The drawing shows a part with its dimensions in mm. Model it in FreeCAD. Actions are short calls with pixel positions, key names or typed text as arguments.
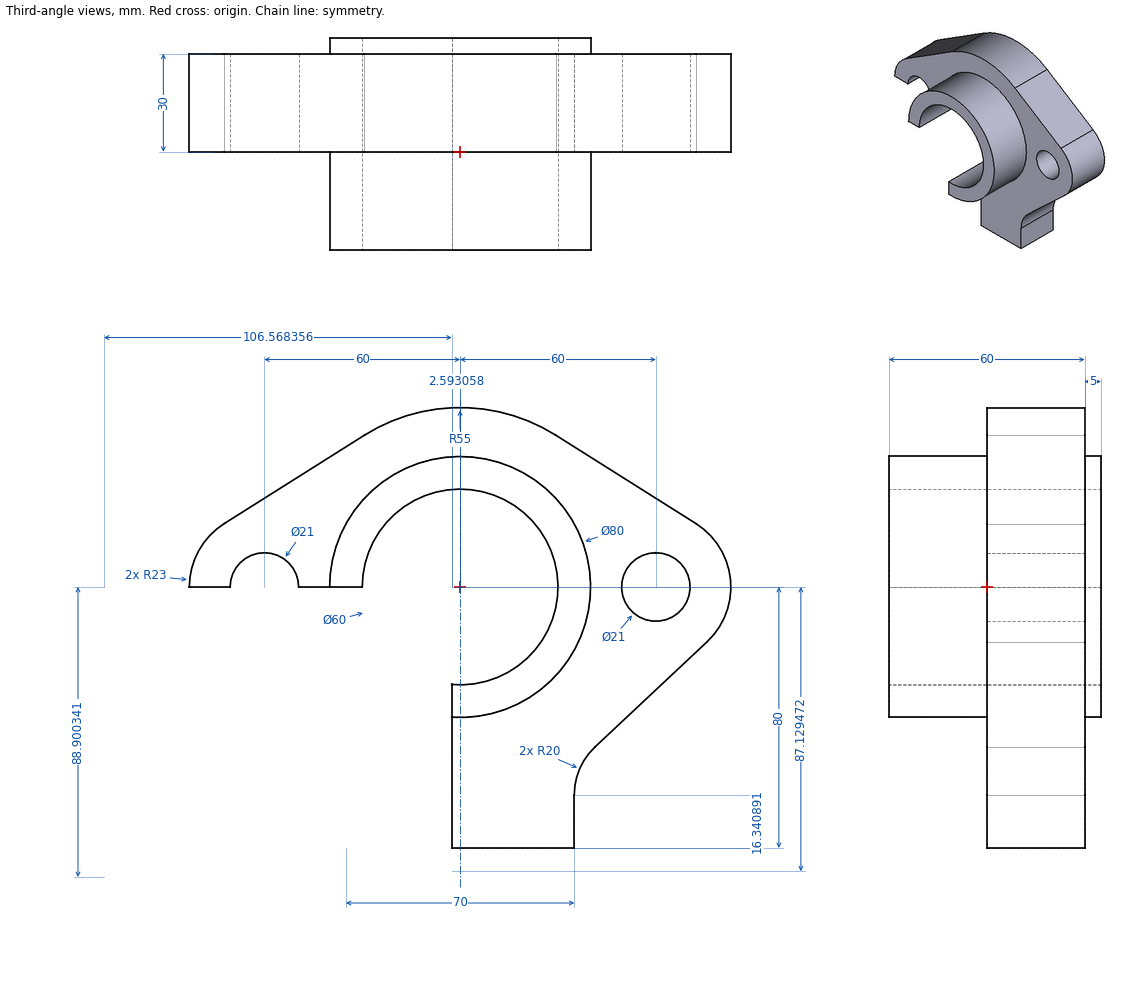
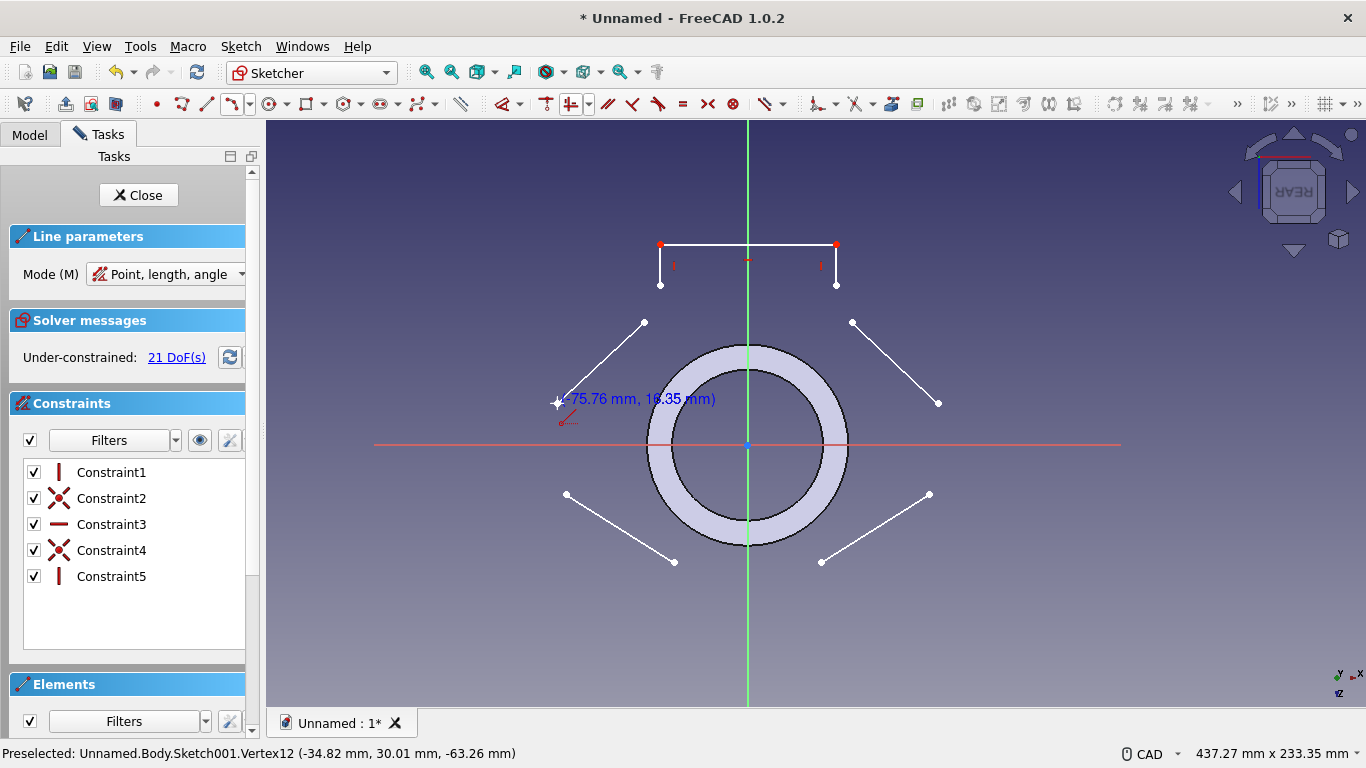
click(232, 104)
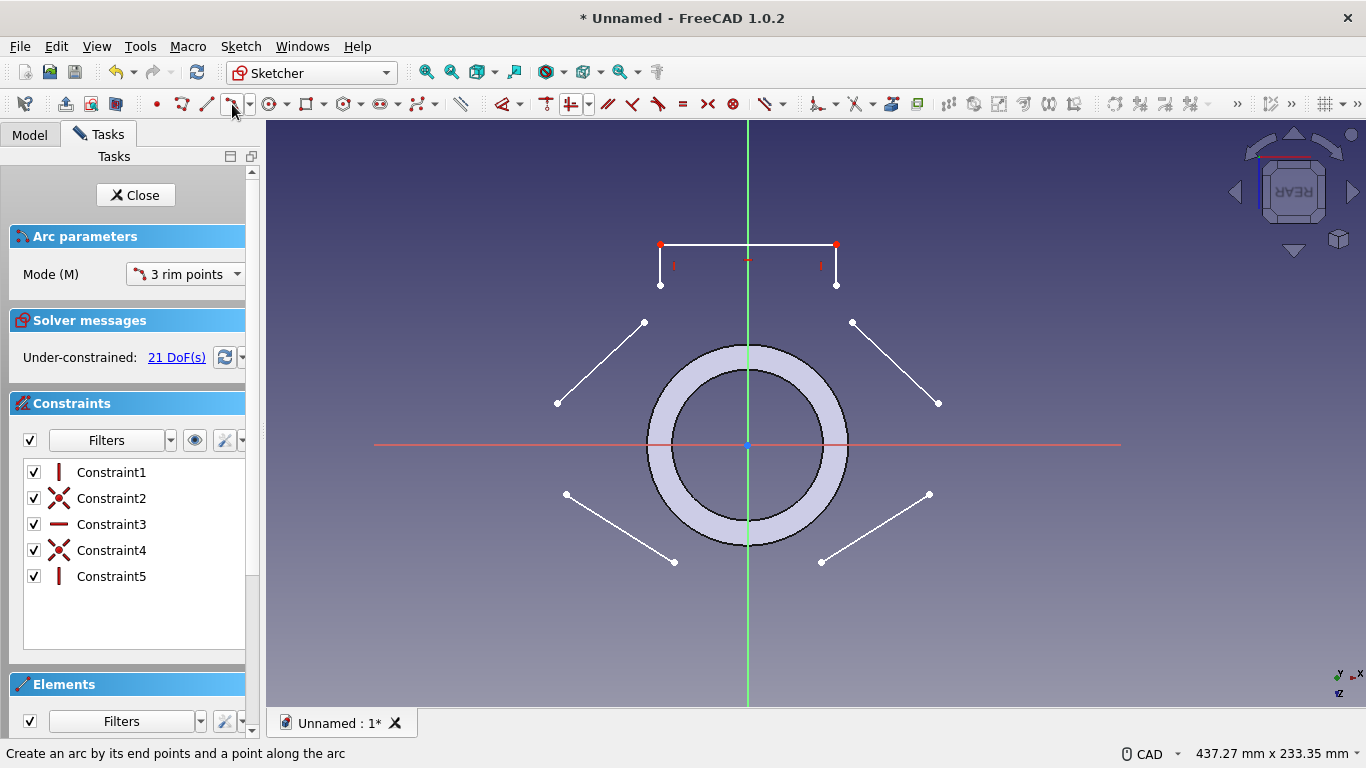
click(674, 563)
click(821, 563)
click(732, 583)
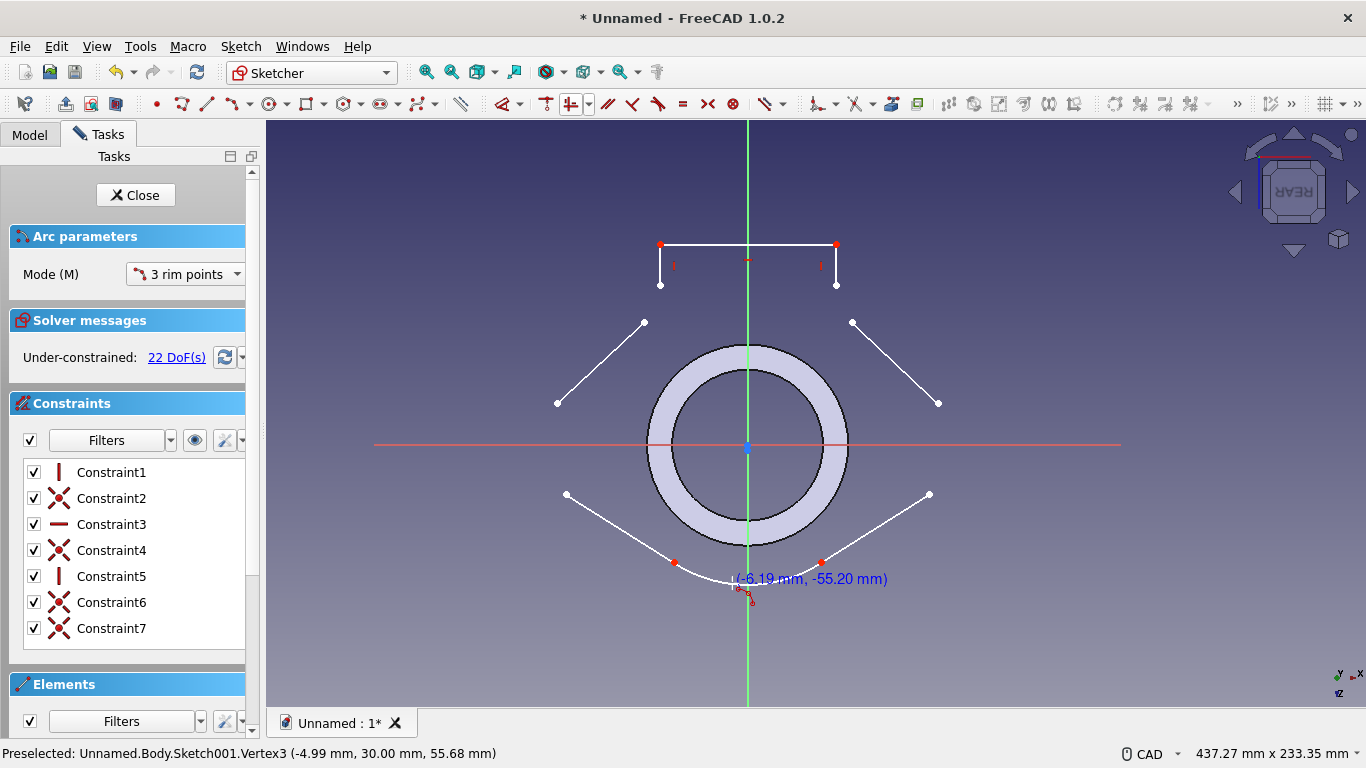
click(929, 495)
click(938, 404)
click(954, 461)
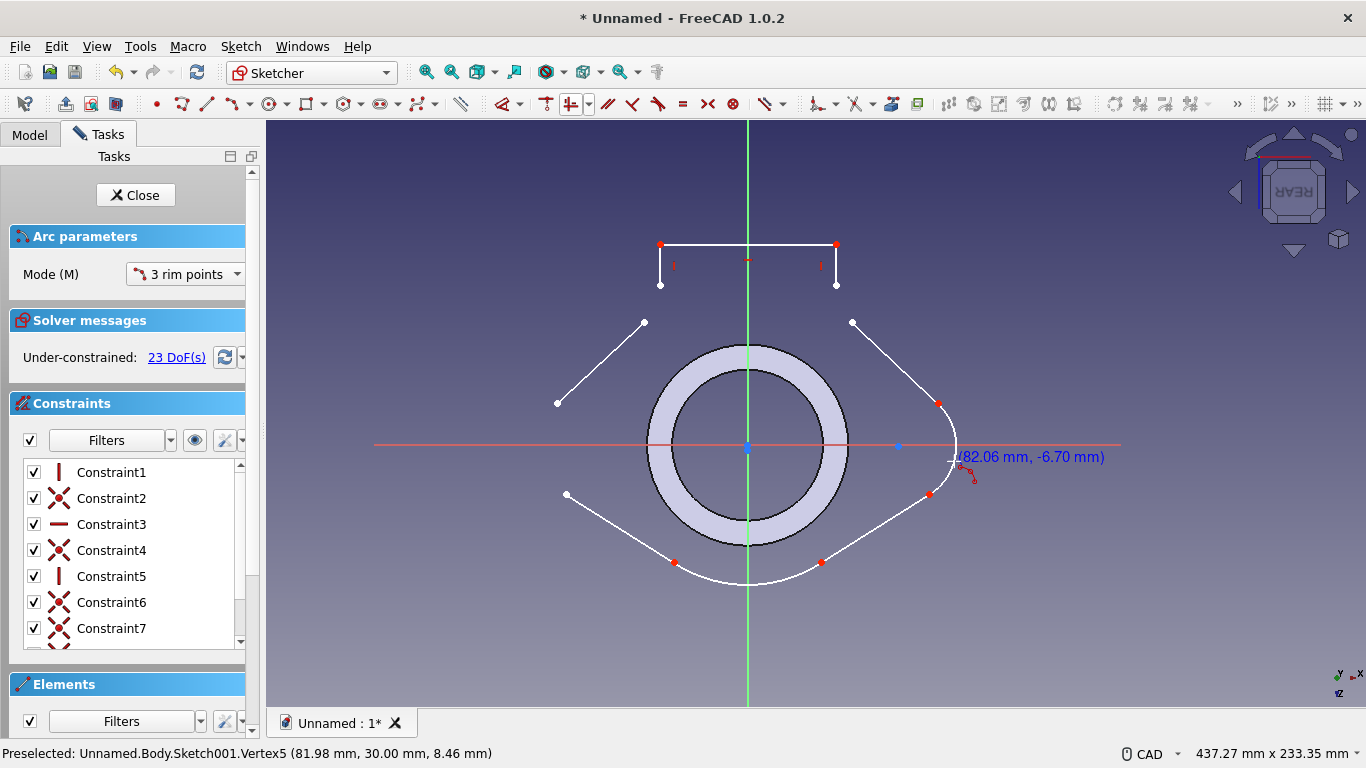
click(852, 323)
click(836, 286)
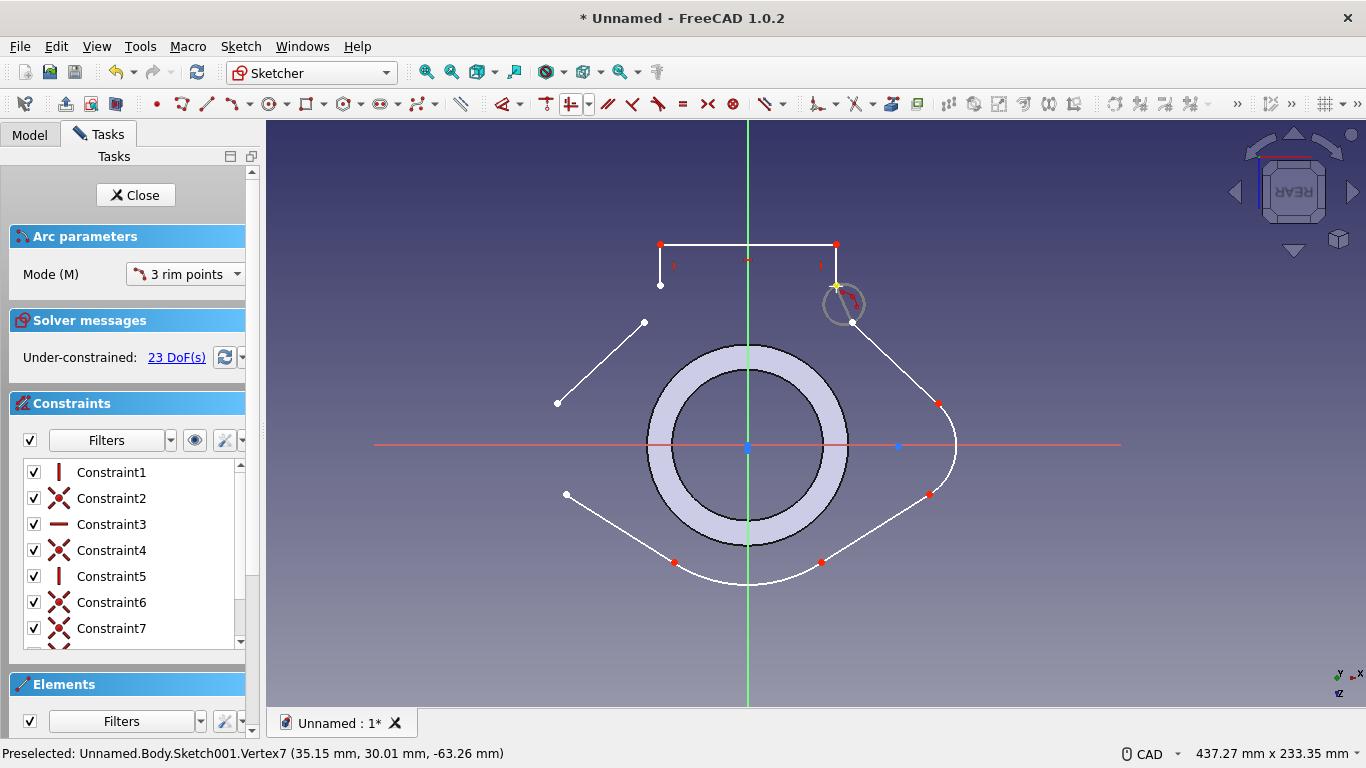
scroll(840, 305, up, 7)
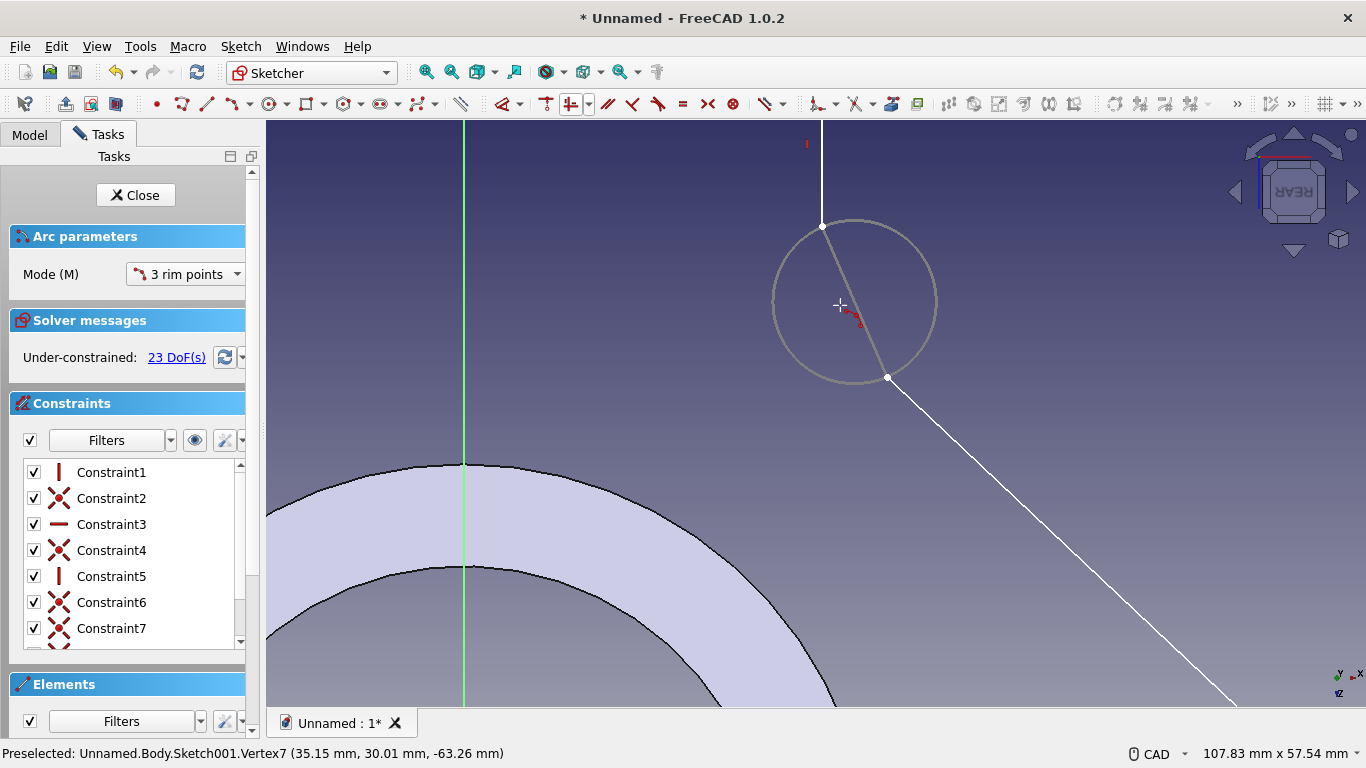
click(837, 304)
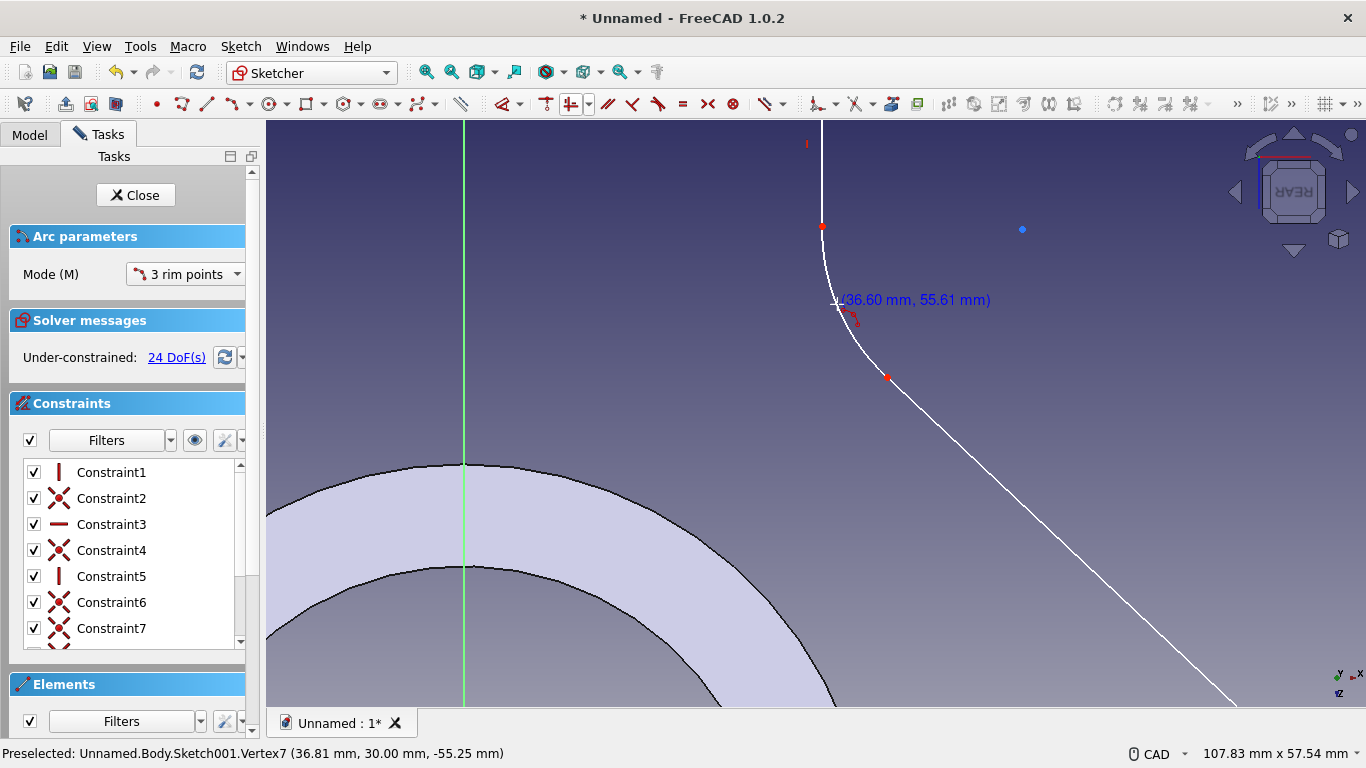
scroll(840, 305, down, 7)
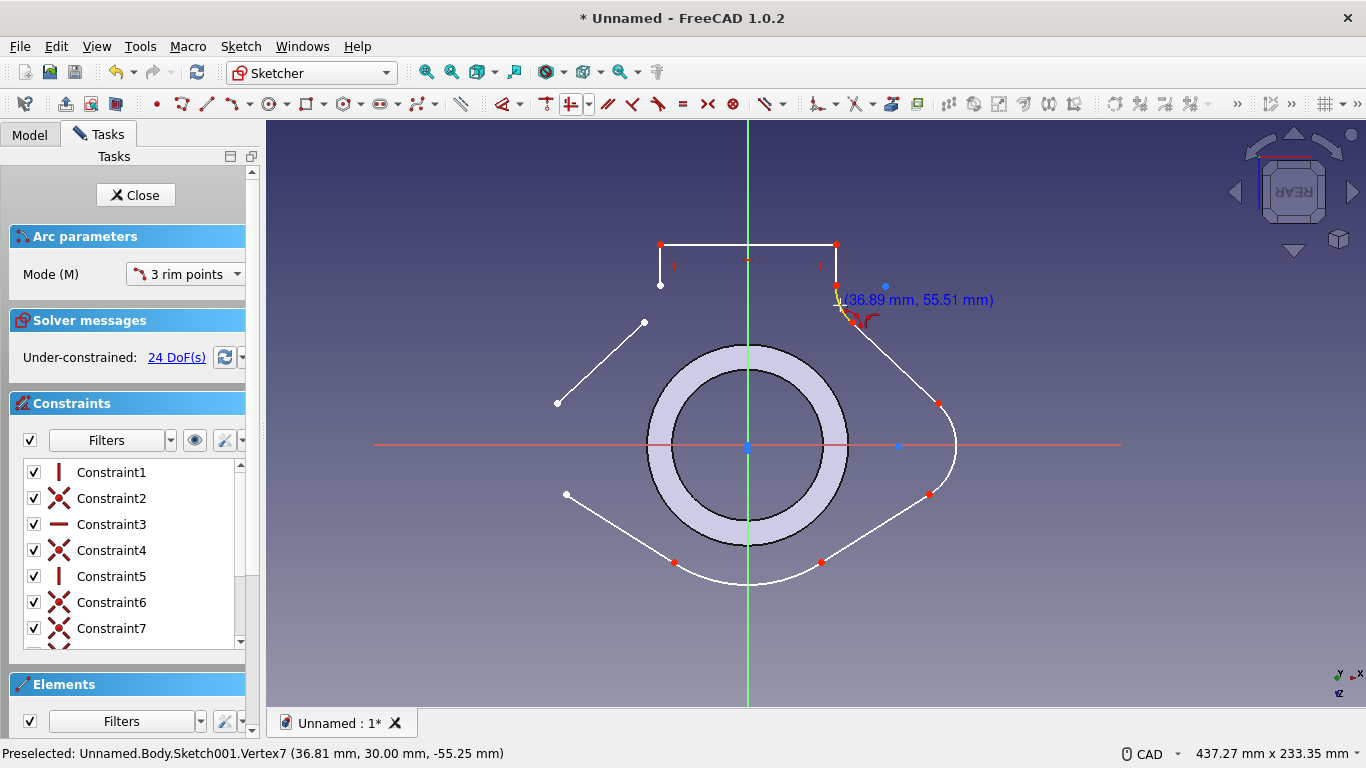
click(660, 286)
click(644, 323)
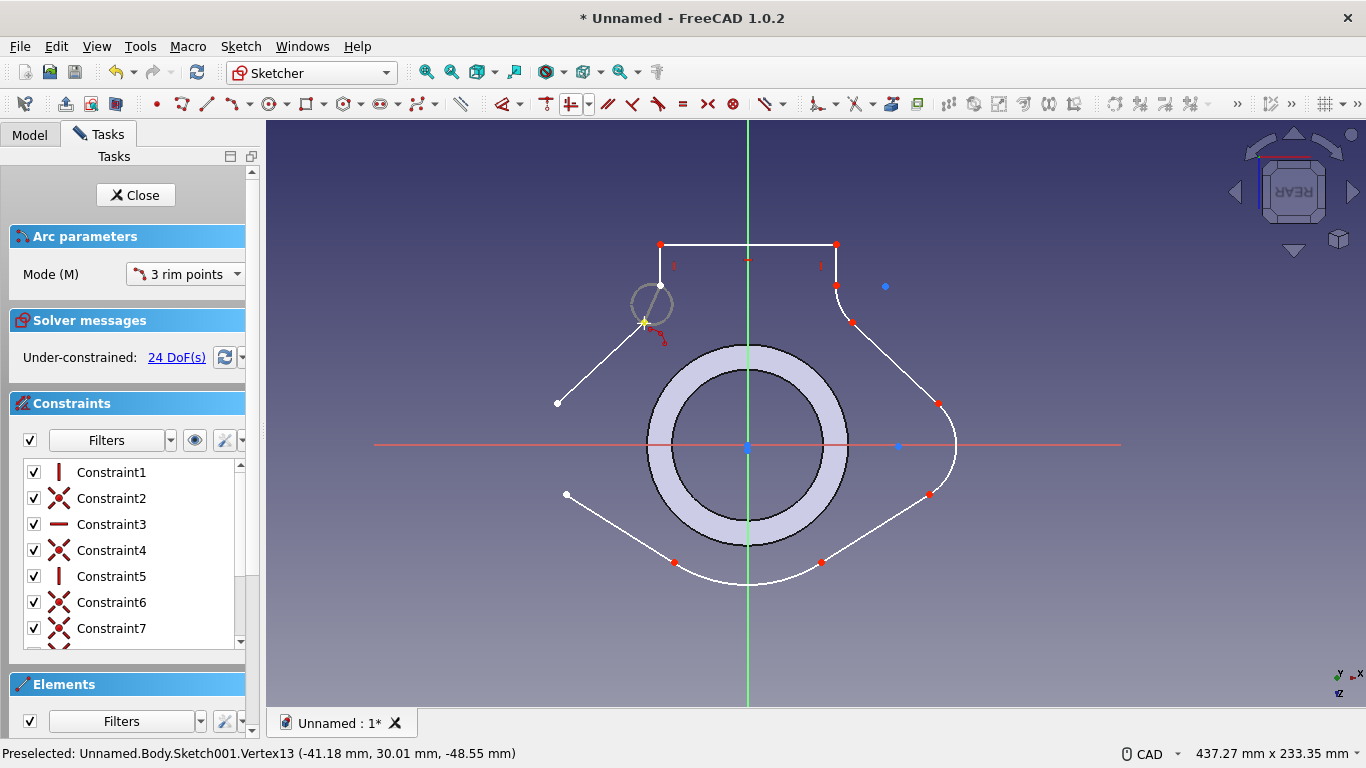
scroll(655, 305, up, 7)